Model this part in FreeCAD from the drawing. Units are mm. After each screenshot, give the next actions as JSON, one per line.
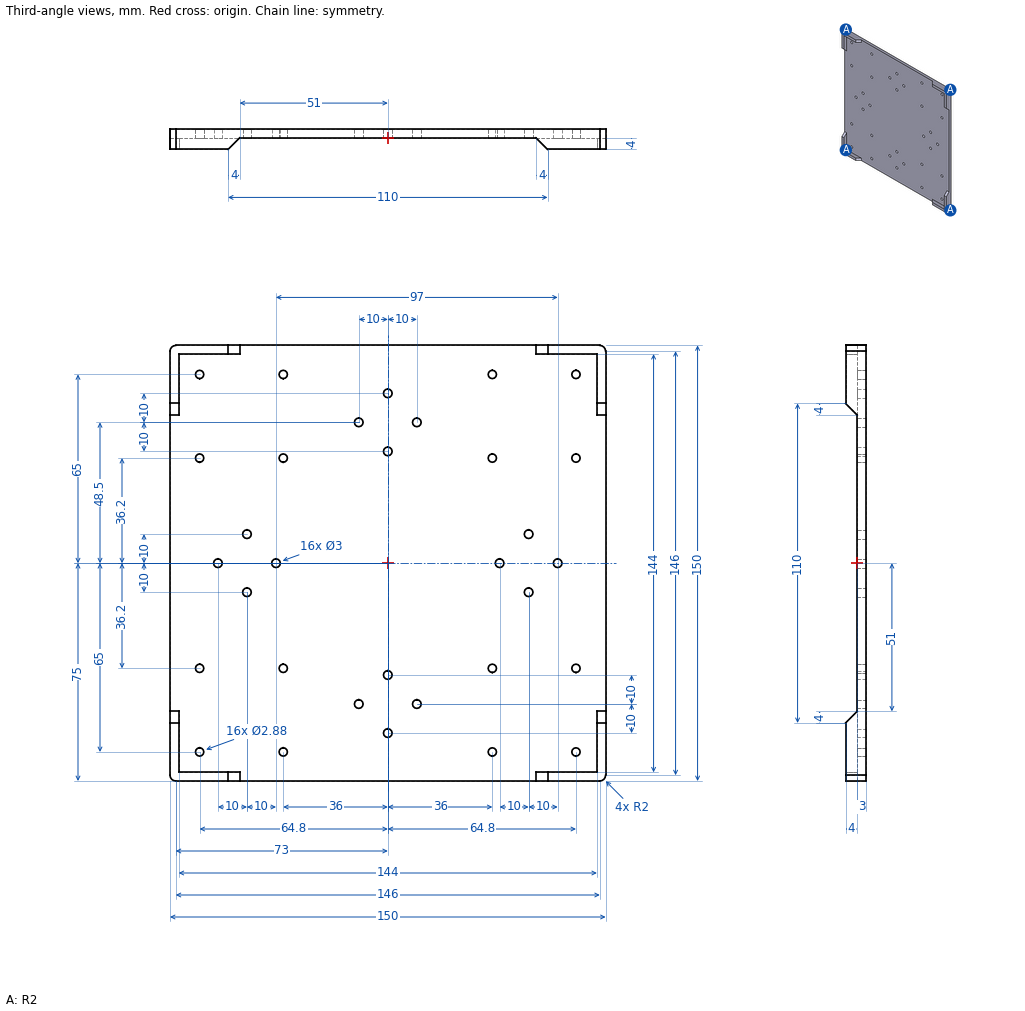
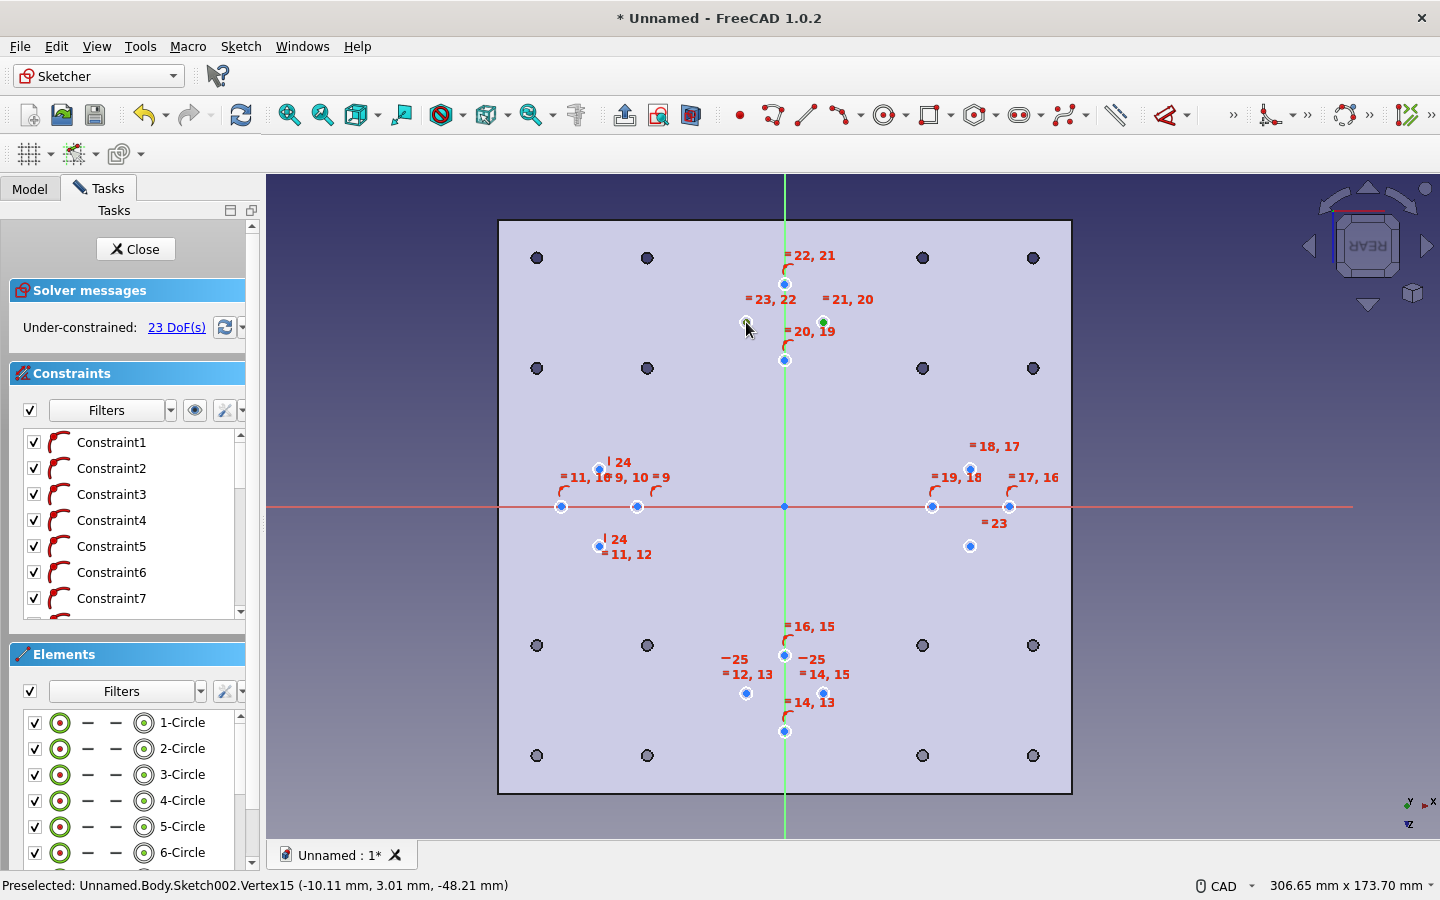
{"action": "key", "text": "h"}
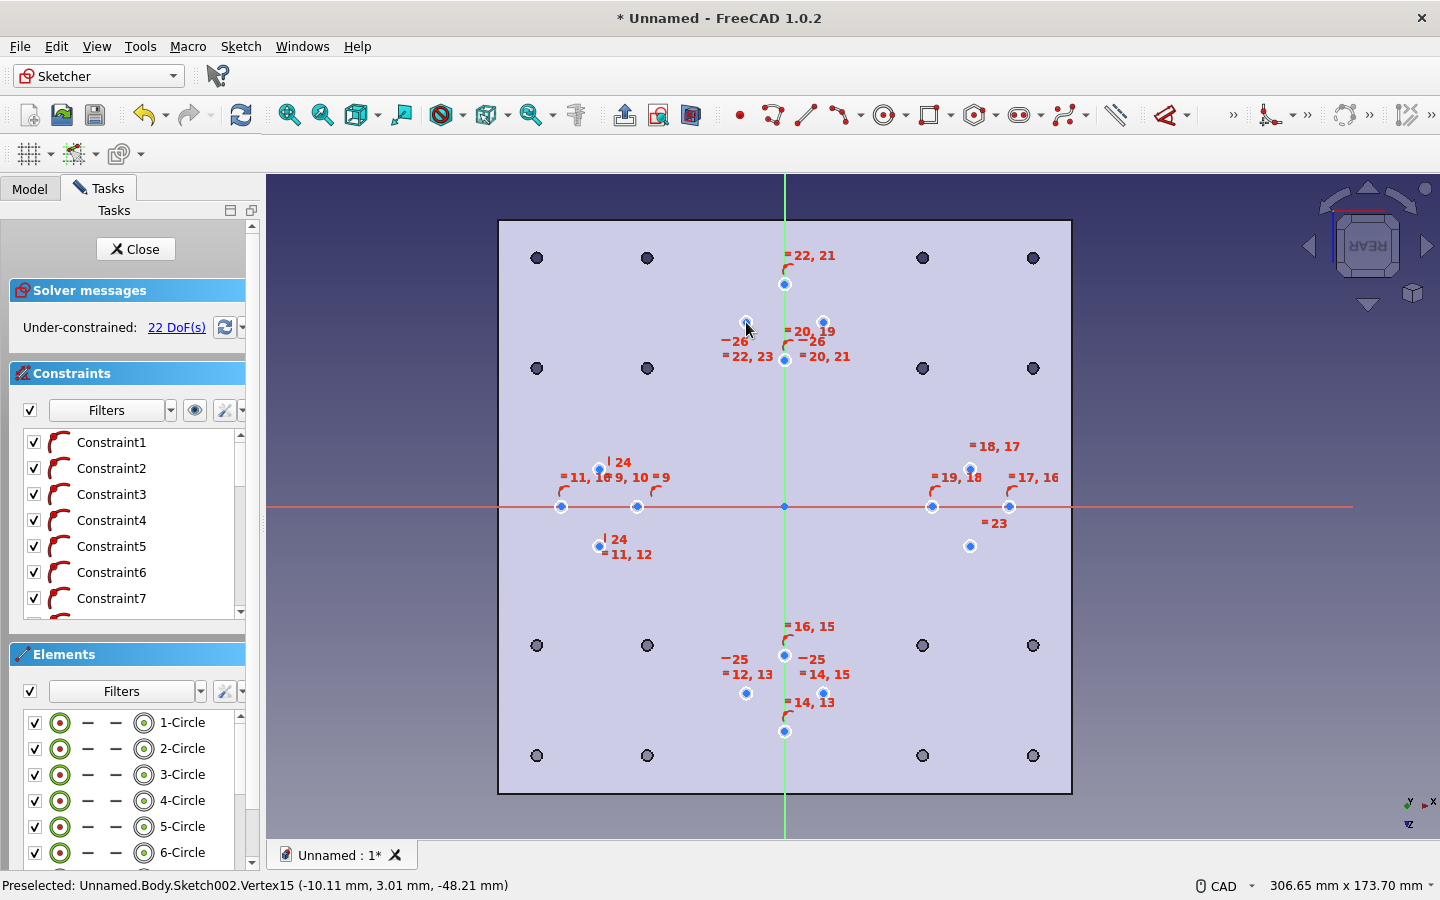
{"action": "left_click", "coordinate": [970, 469]}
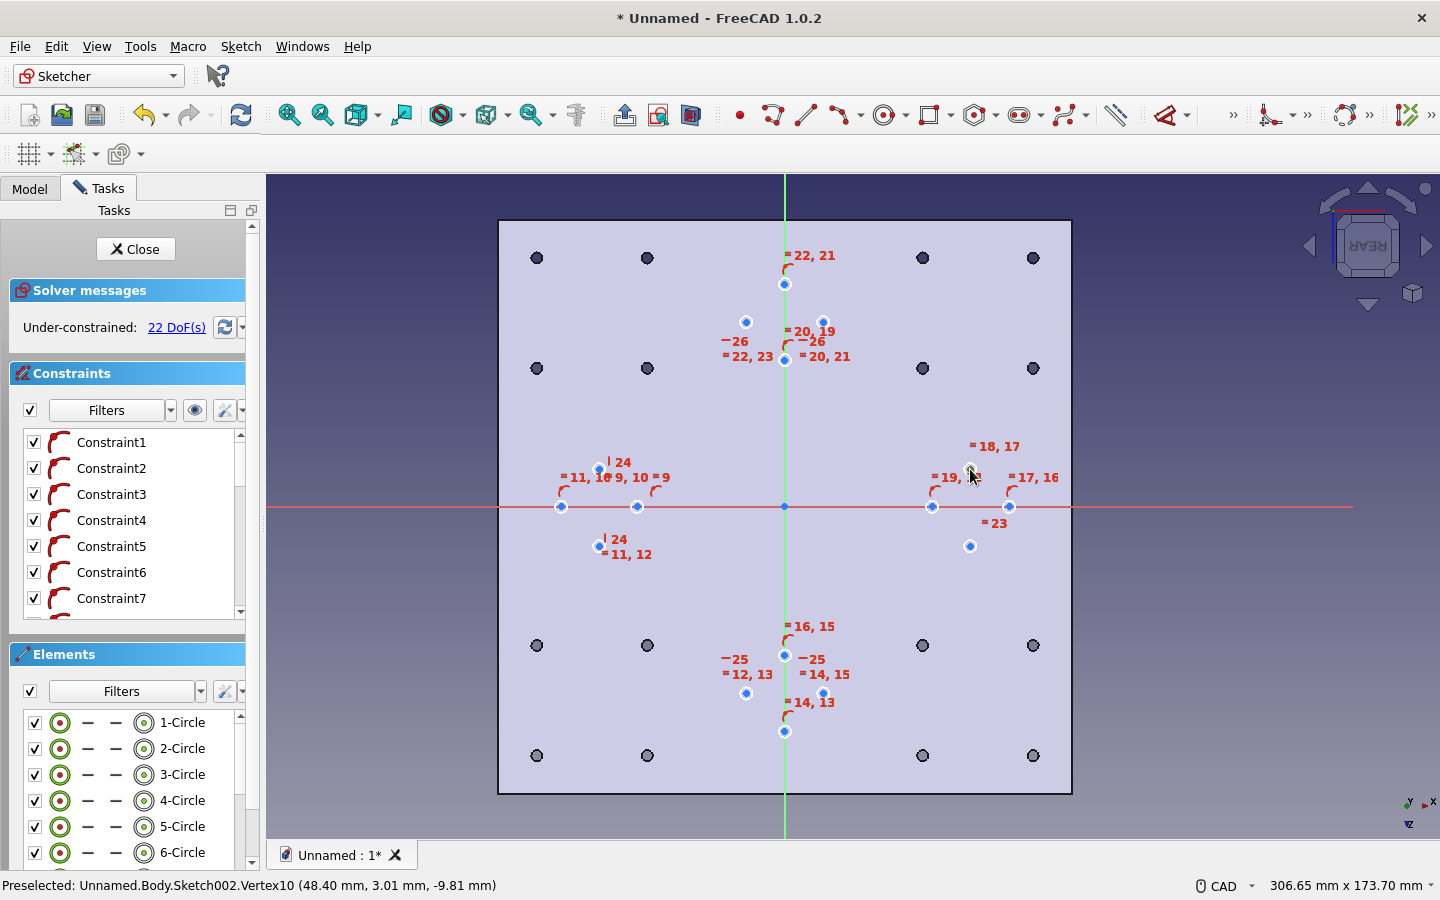
{"action": "left_click", "coordinate": [970, 546]}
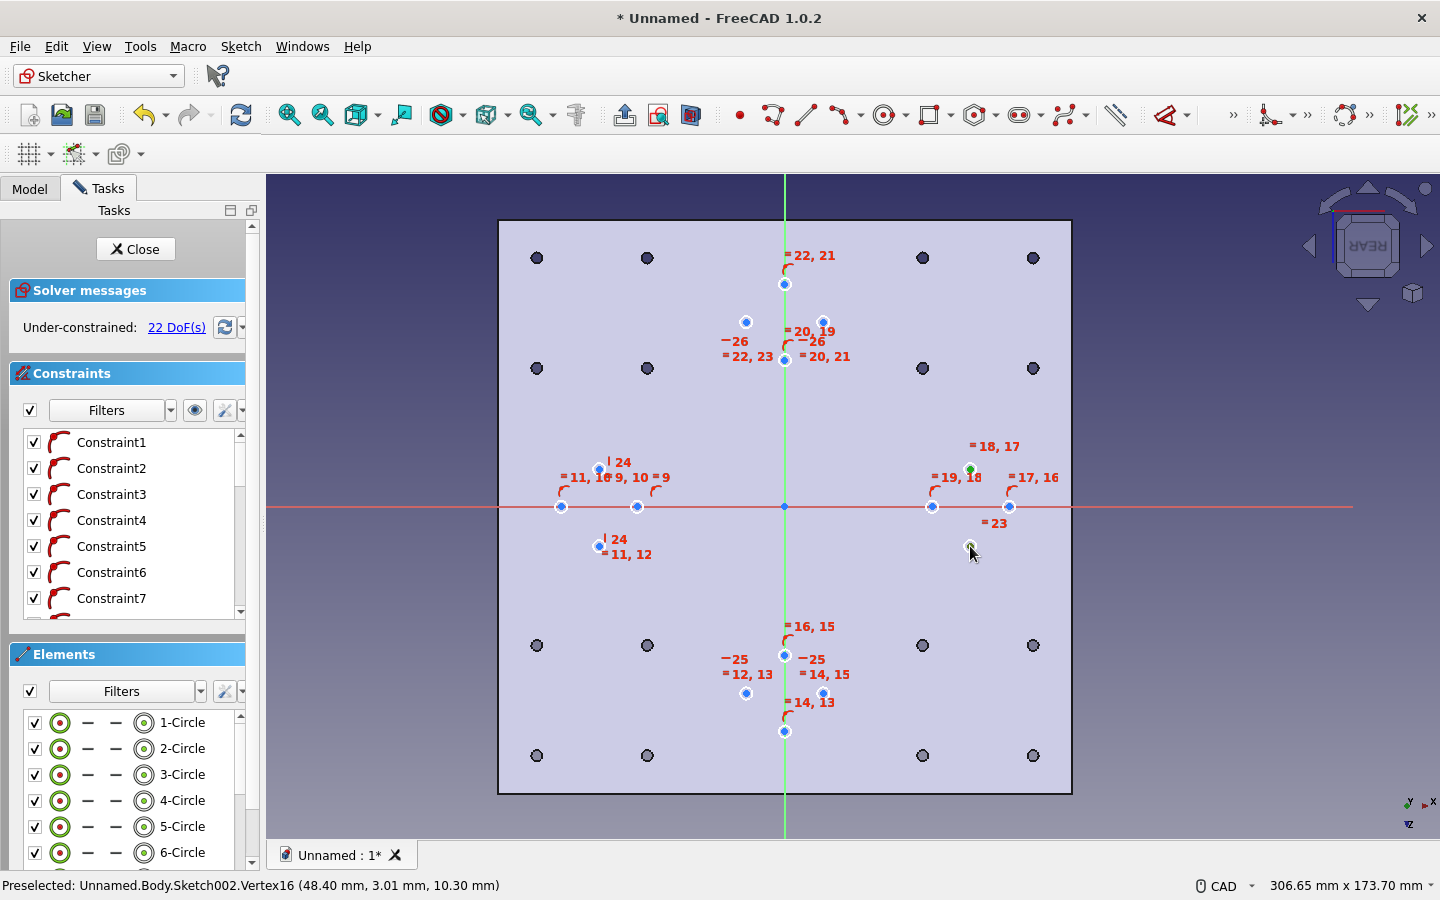
{"action": "key", "text": "v"}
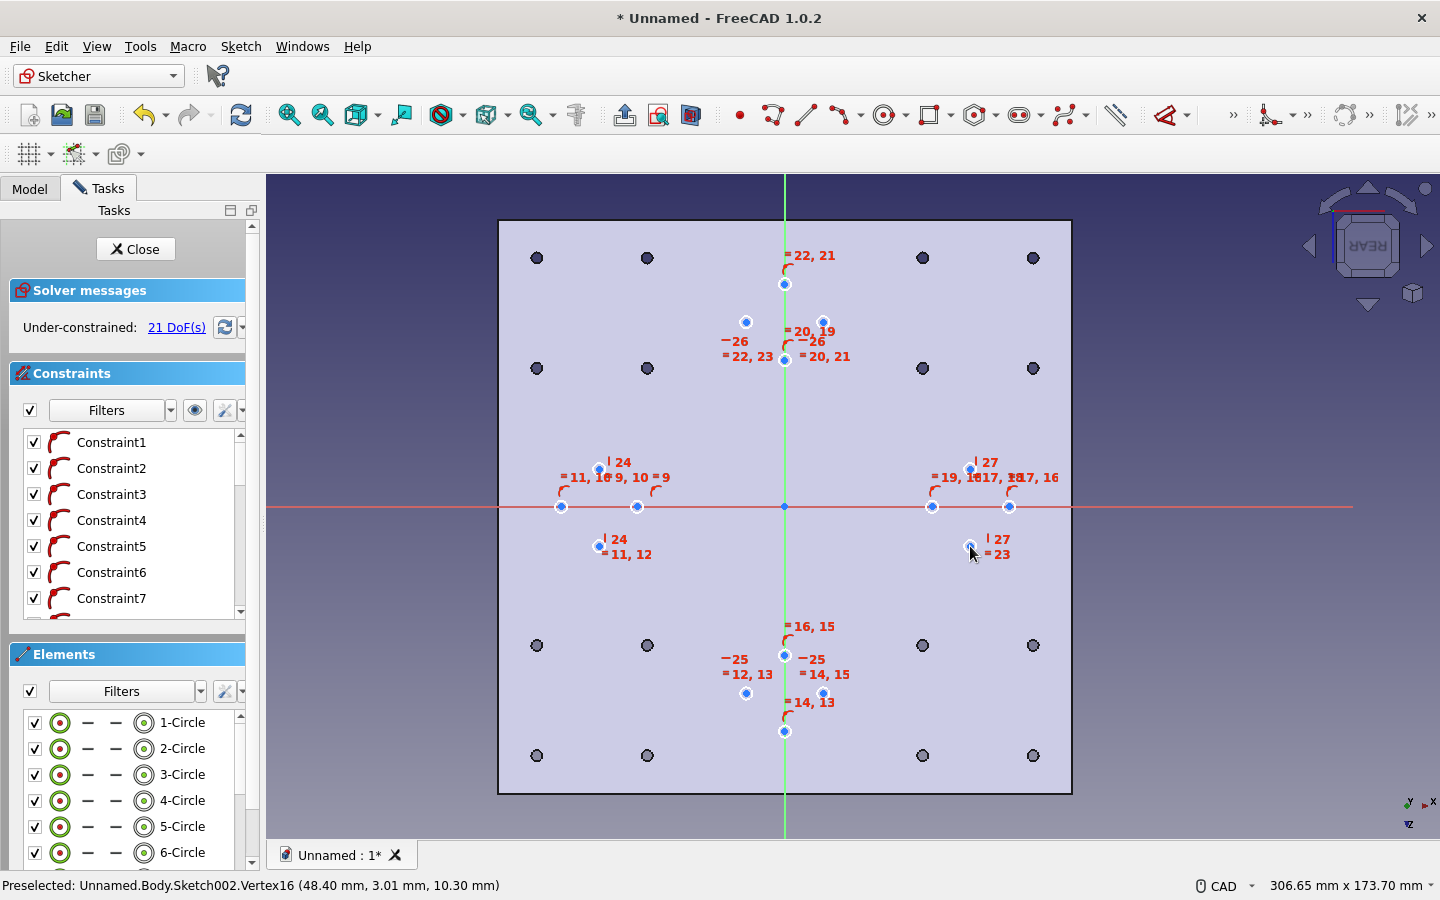
{"action": "left_click", "coordinate": [599, 469]}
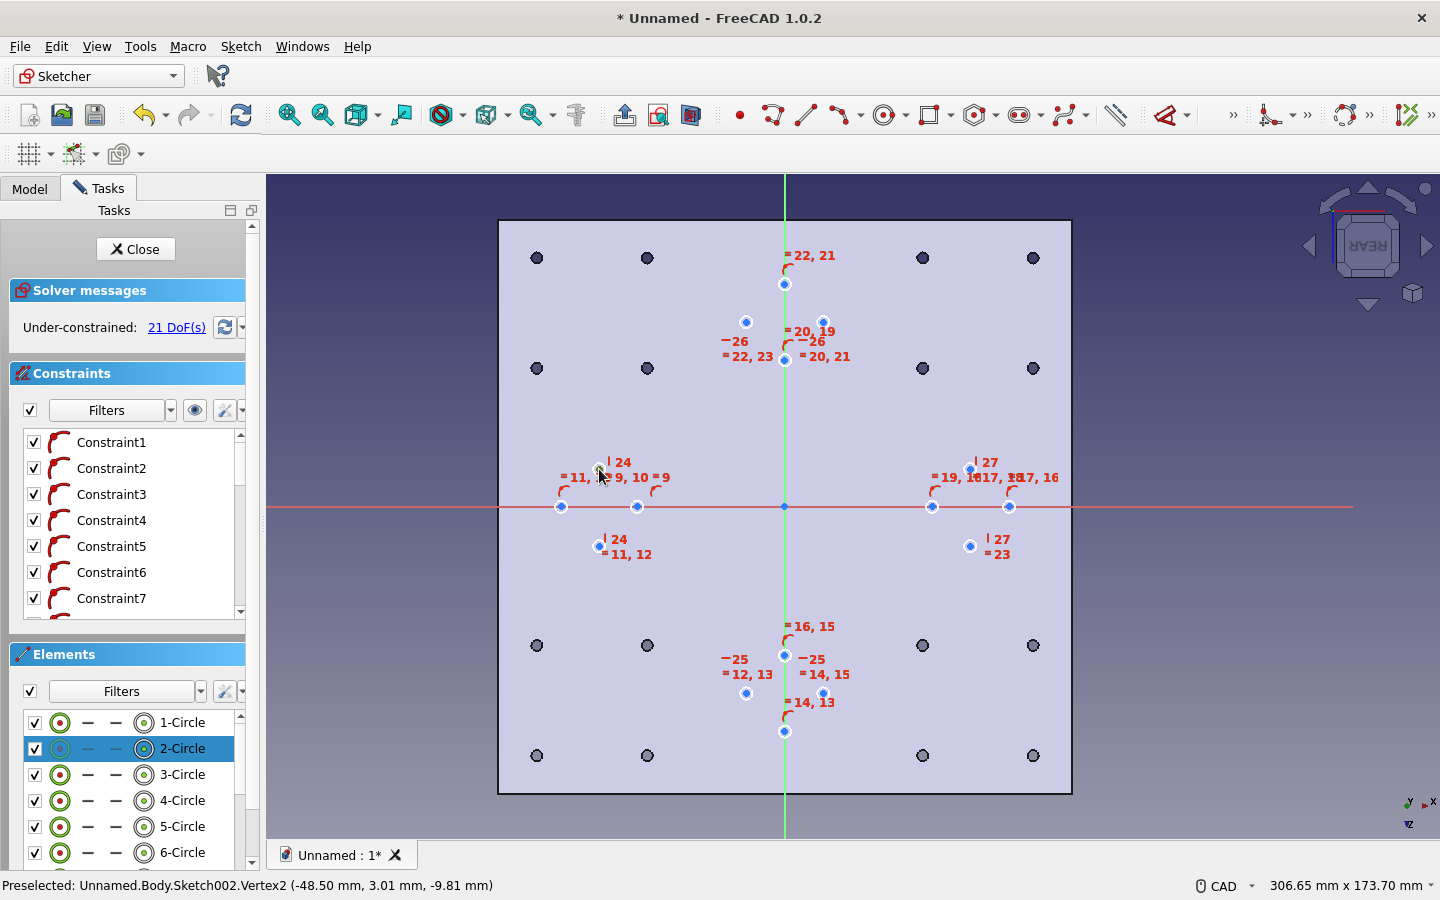
{"action": "left_click", "coordinate": [970, 469]}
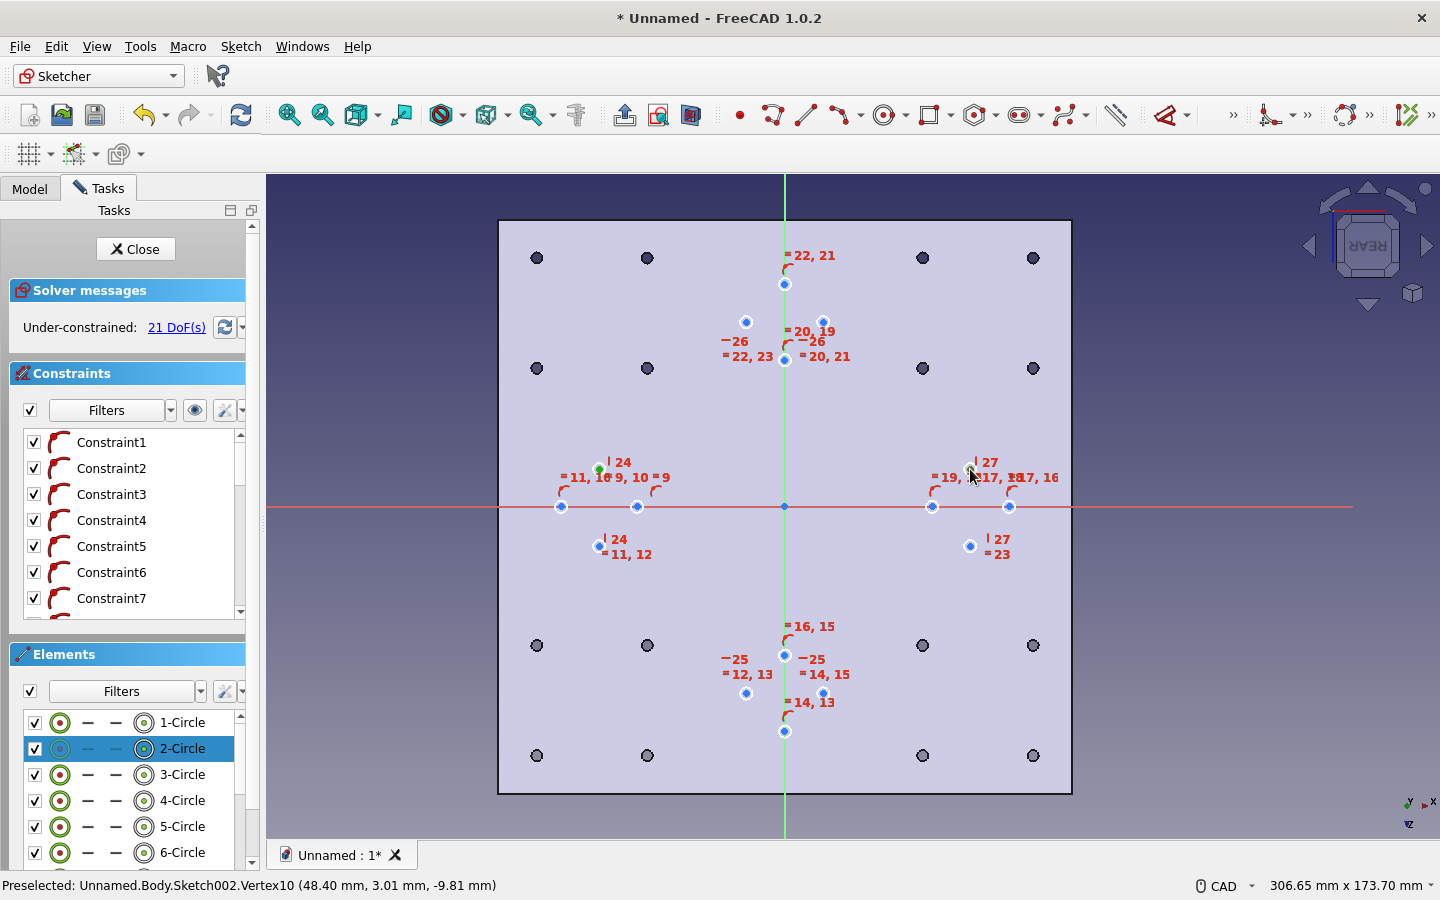
{"action": "left_click", "coordinate": [785, 594]}